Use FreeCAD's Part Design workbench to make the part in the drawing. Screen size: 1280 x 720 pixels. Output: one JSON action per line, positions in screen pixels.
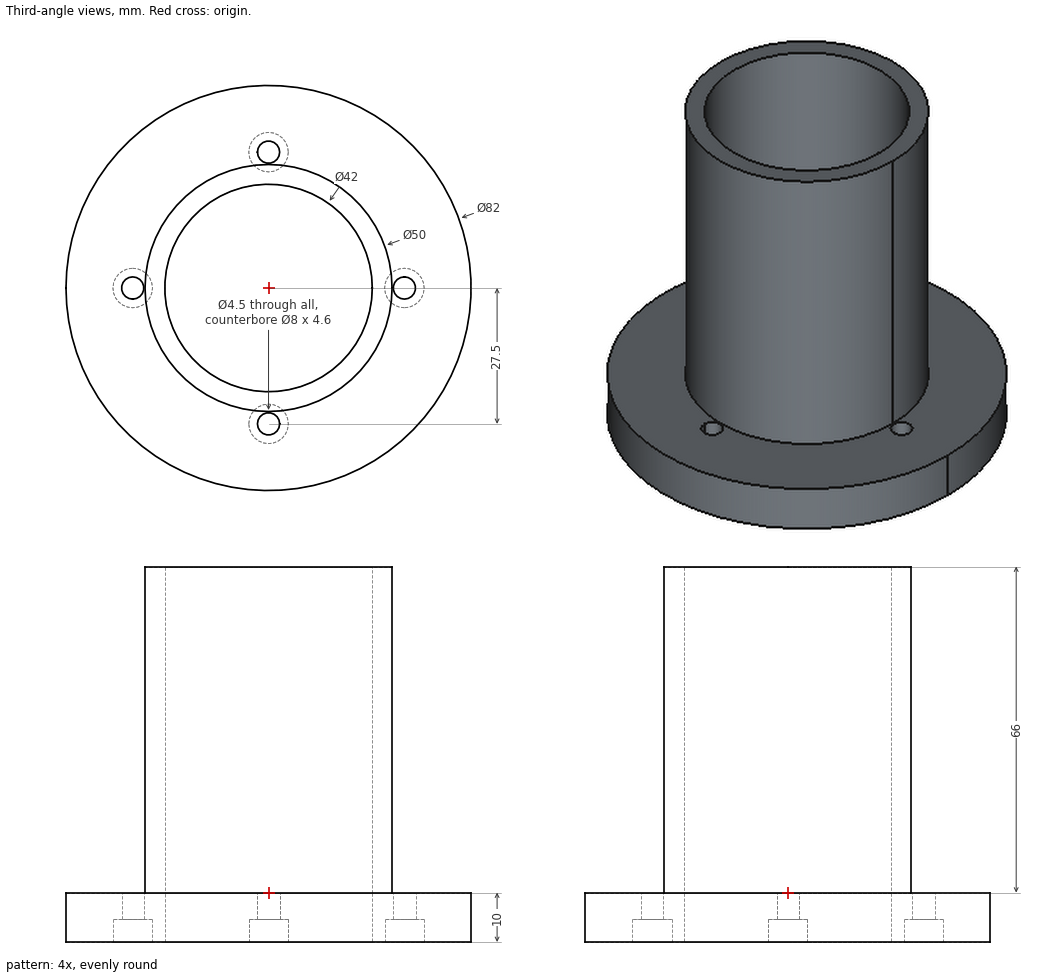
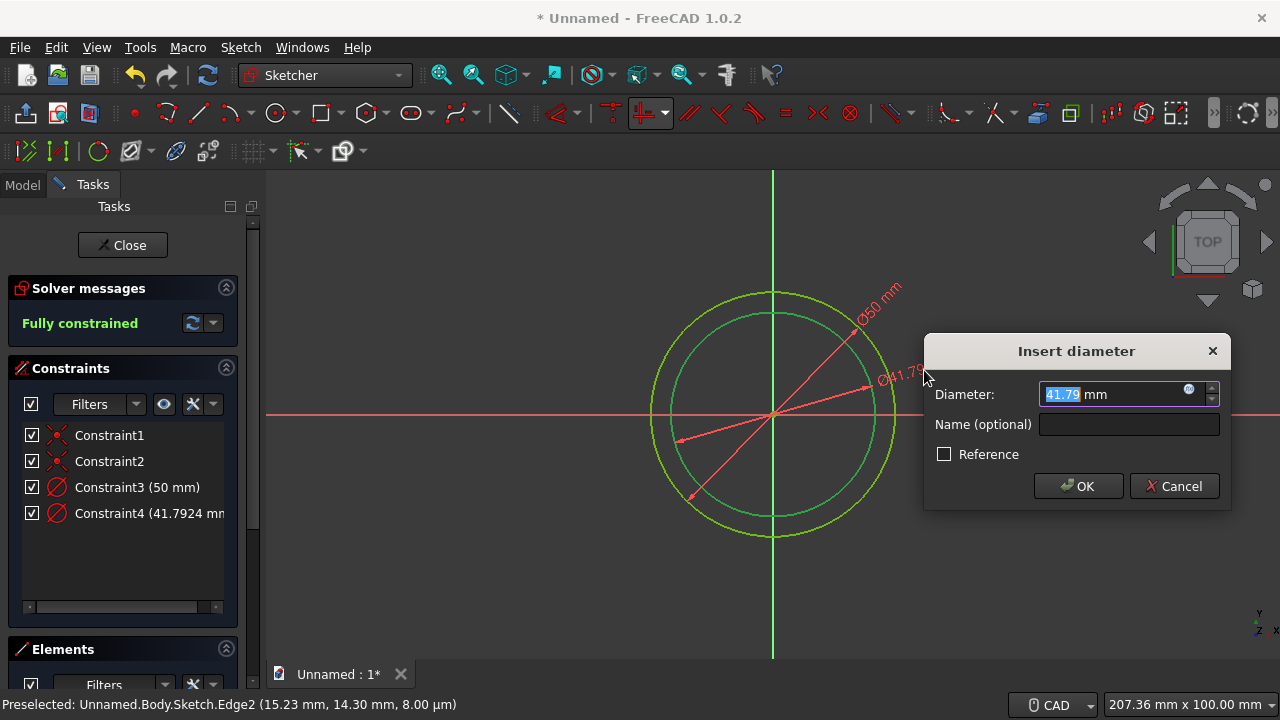
{"action": "type", "text": "42"}
{"action": "key", "text": "Return"}
{"action": "key", "text": "Escape"}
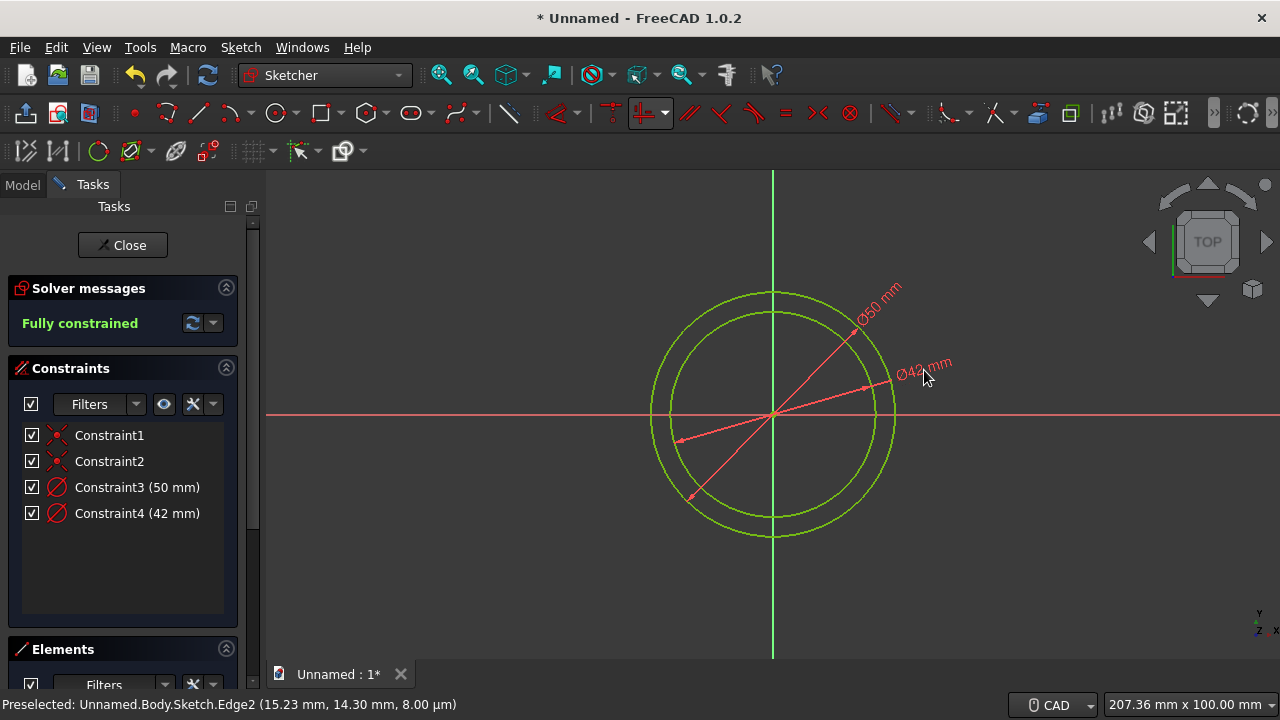
{"action": "left_click", "coordinate": [123, 245]}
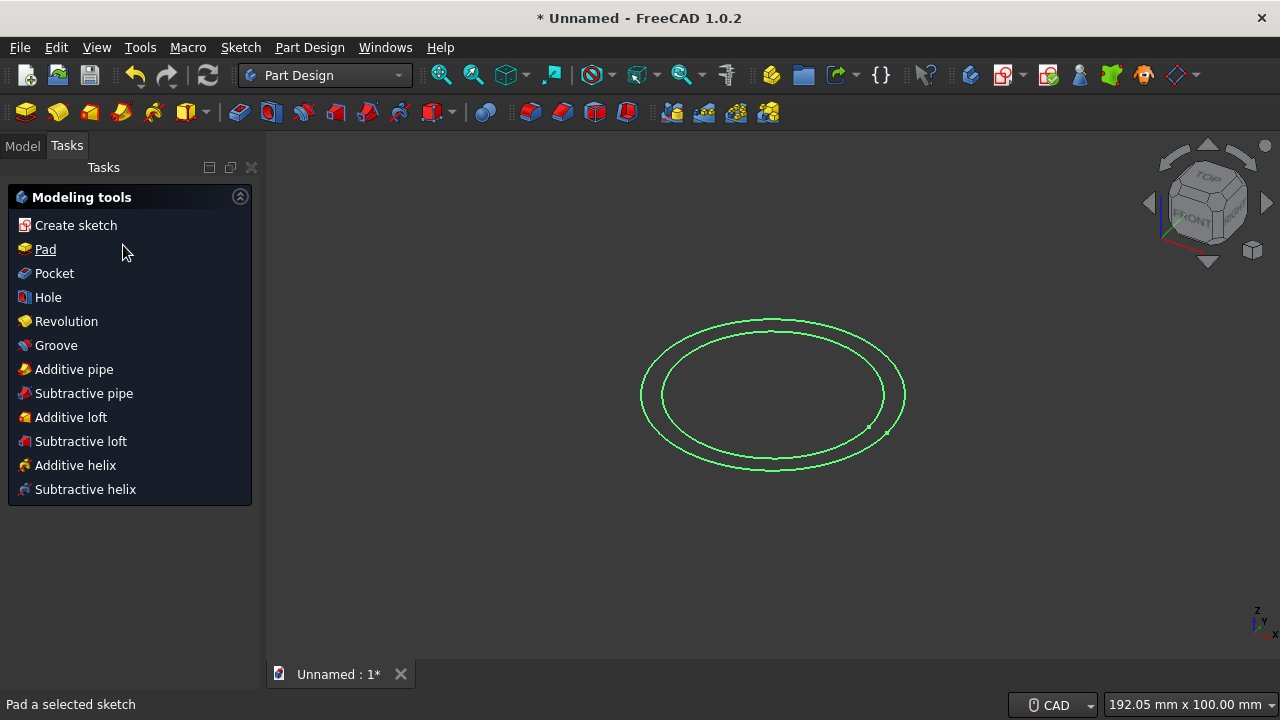
{"action": "left_click", "coordinate": [26, 112]}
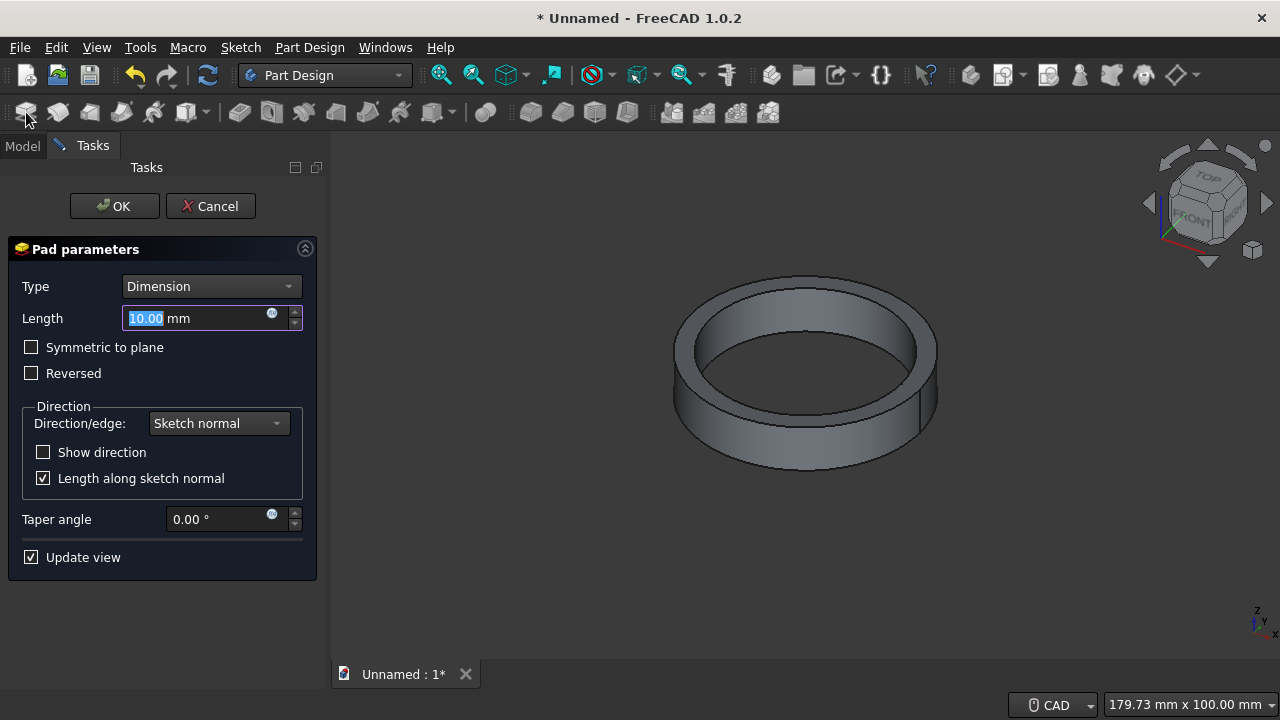
{"action": "type", "text": "66"}
{"action": "key", "text": "Tab"}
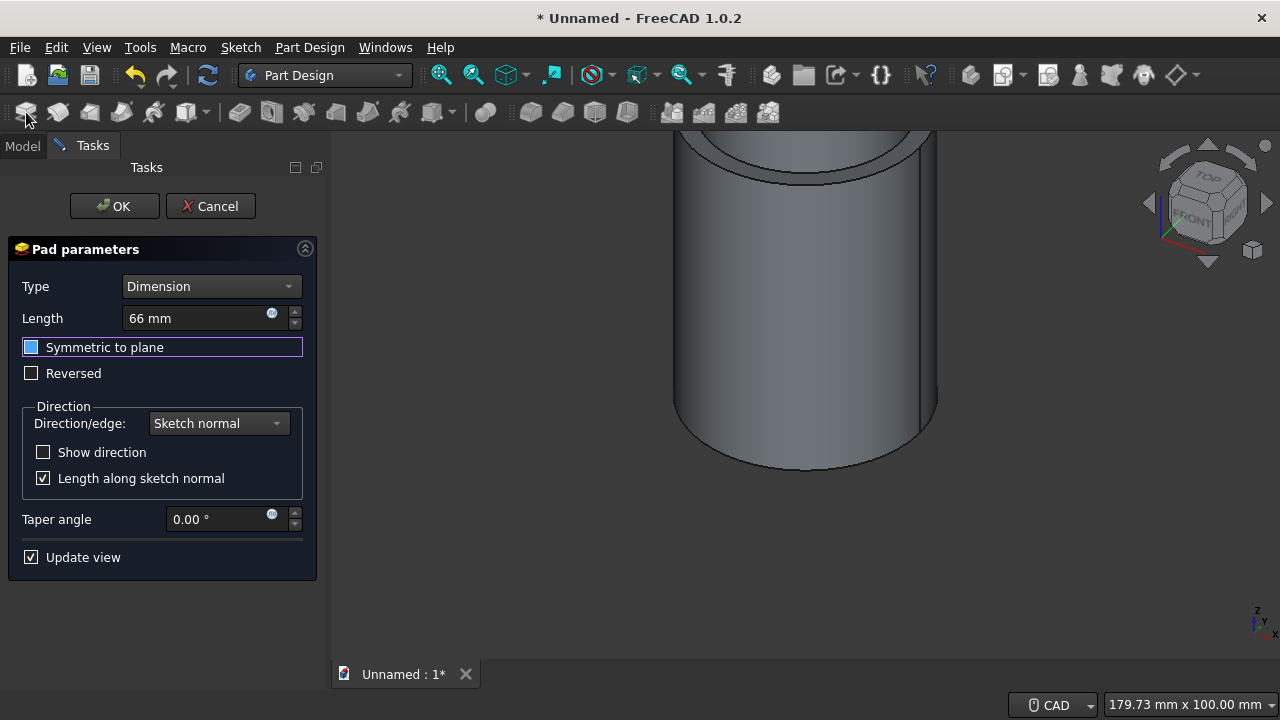
{"action": "left_click", "coordinate": [115, 206]}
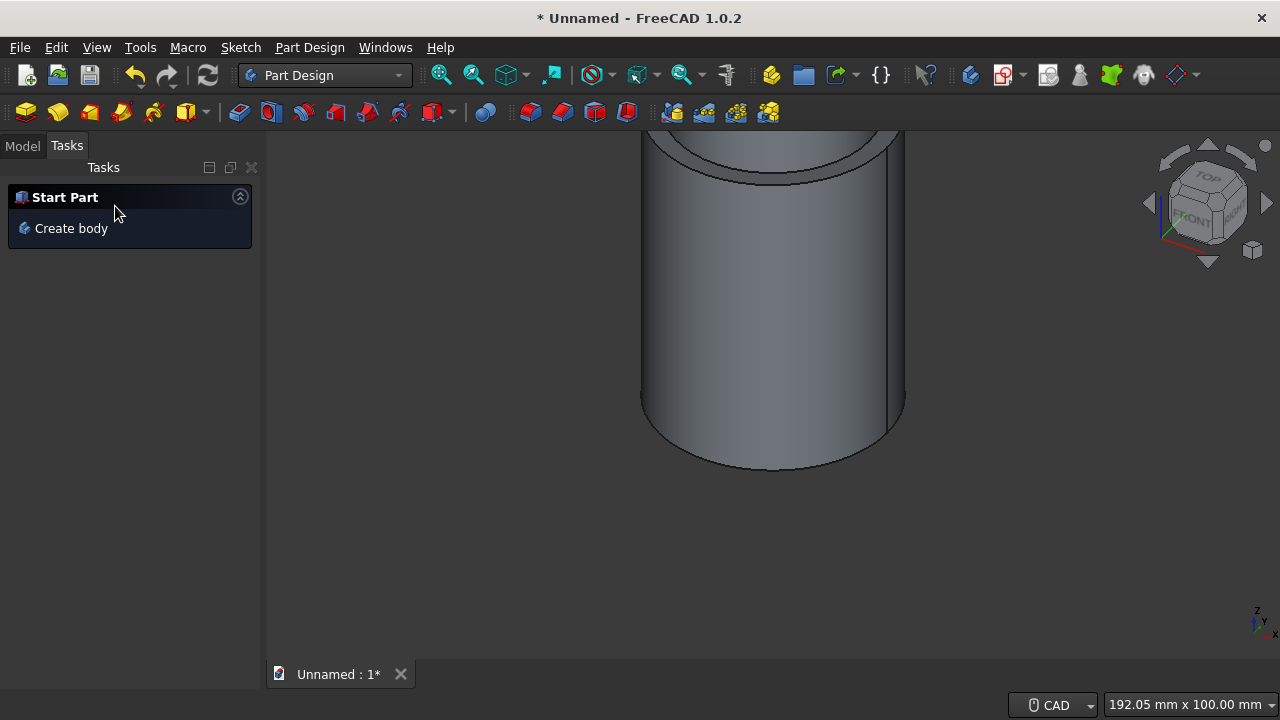
{"action": "left_click", "coordinate": [442, 76]}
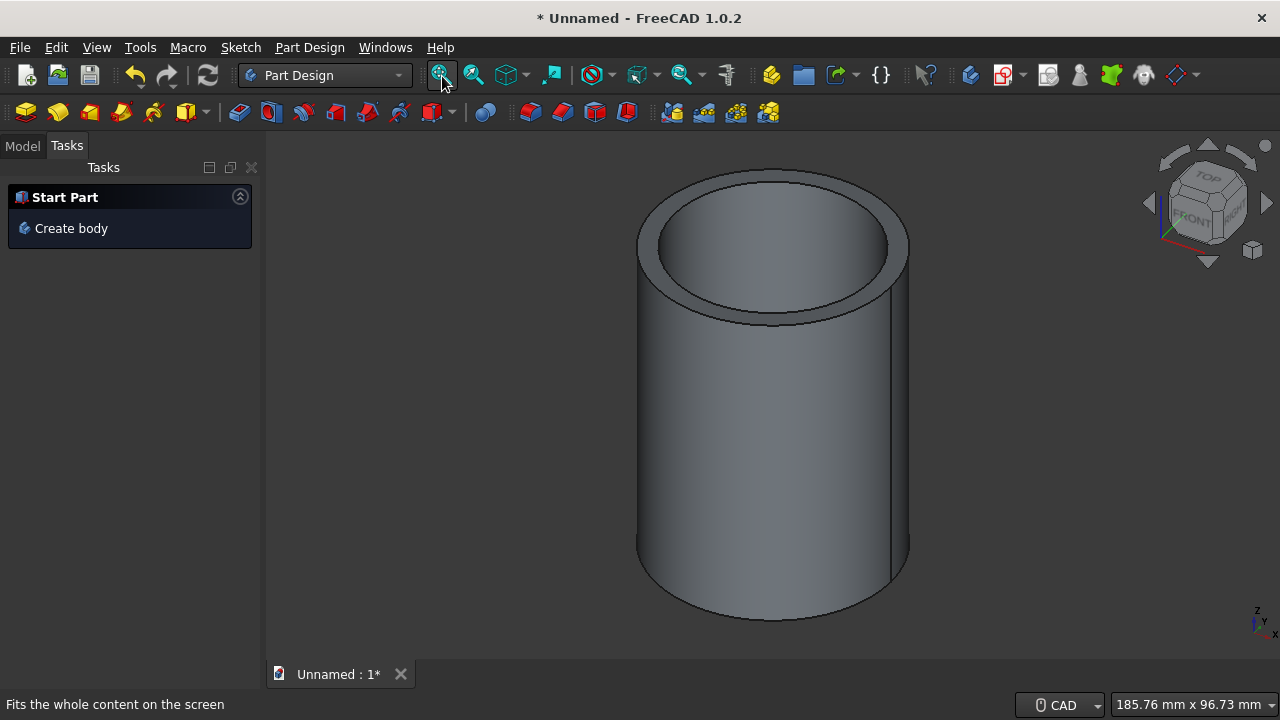
{"action": "left_click", "coordinate": [23, 145]}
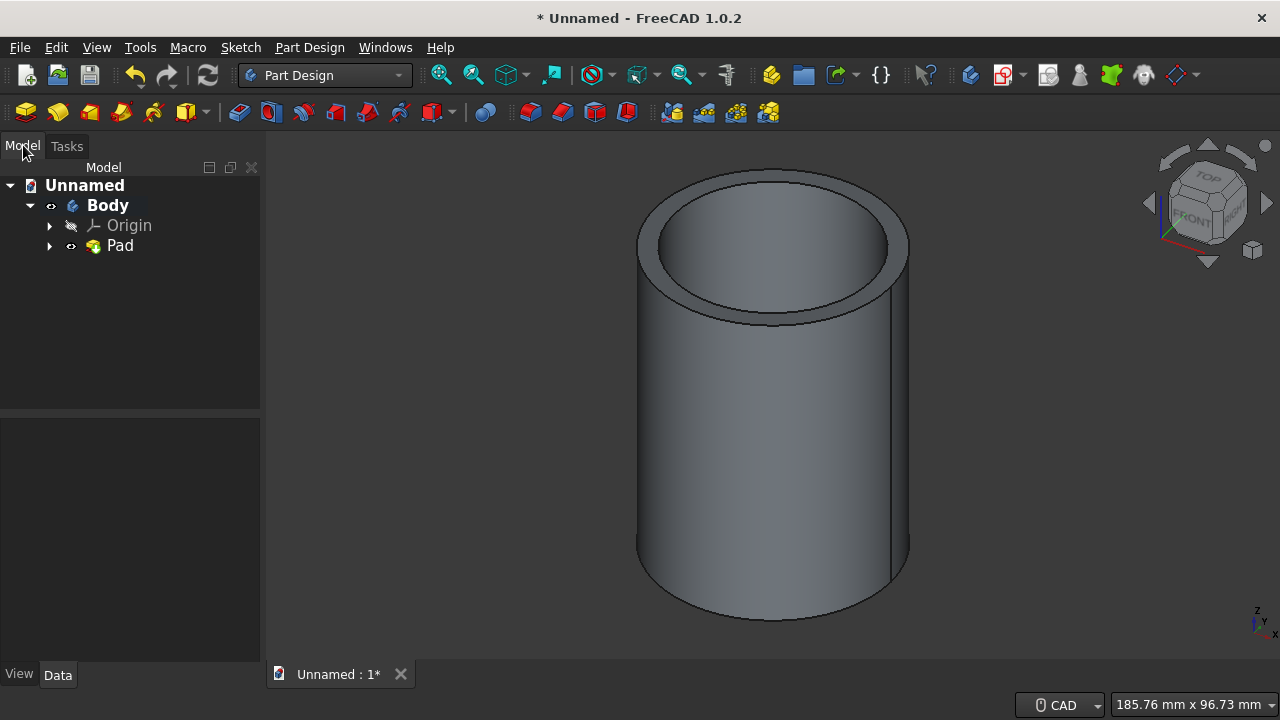
{"action": "left_click", "coordinate": [50, 226]}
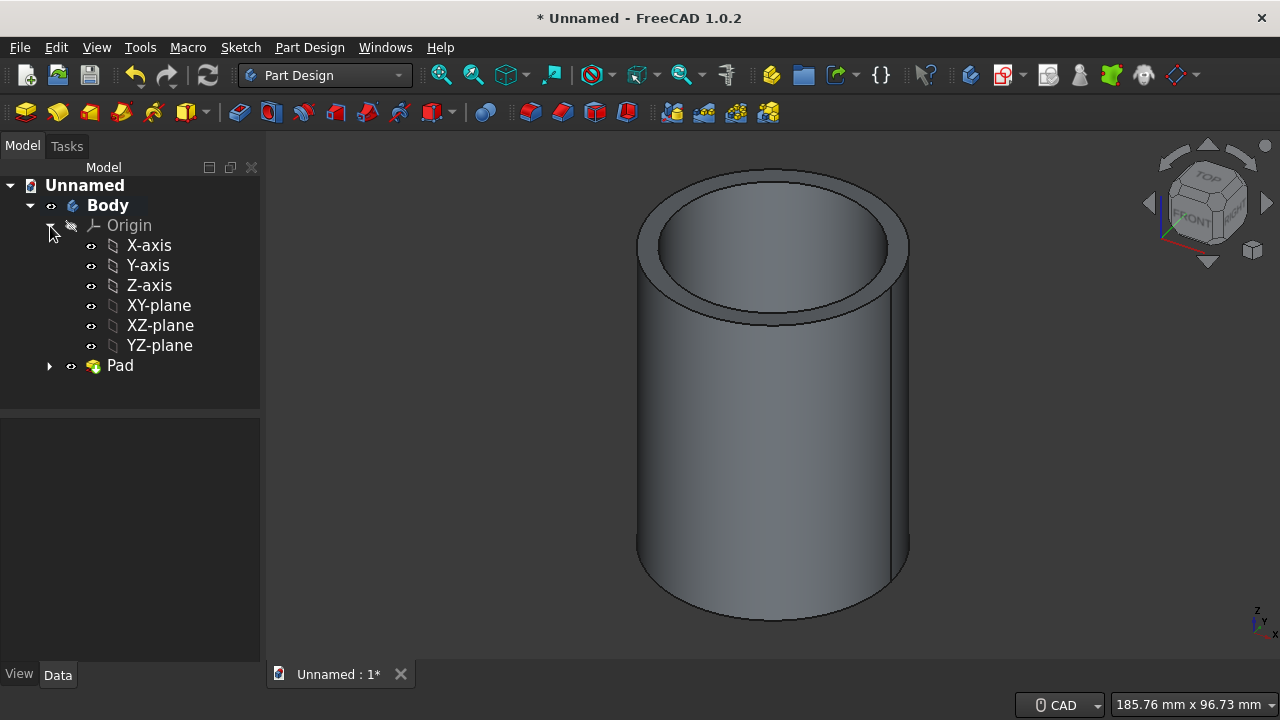
{"action": "left_click", "coordinate": [136, 306]}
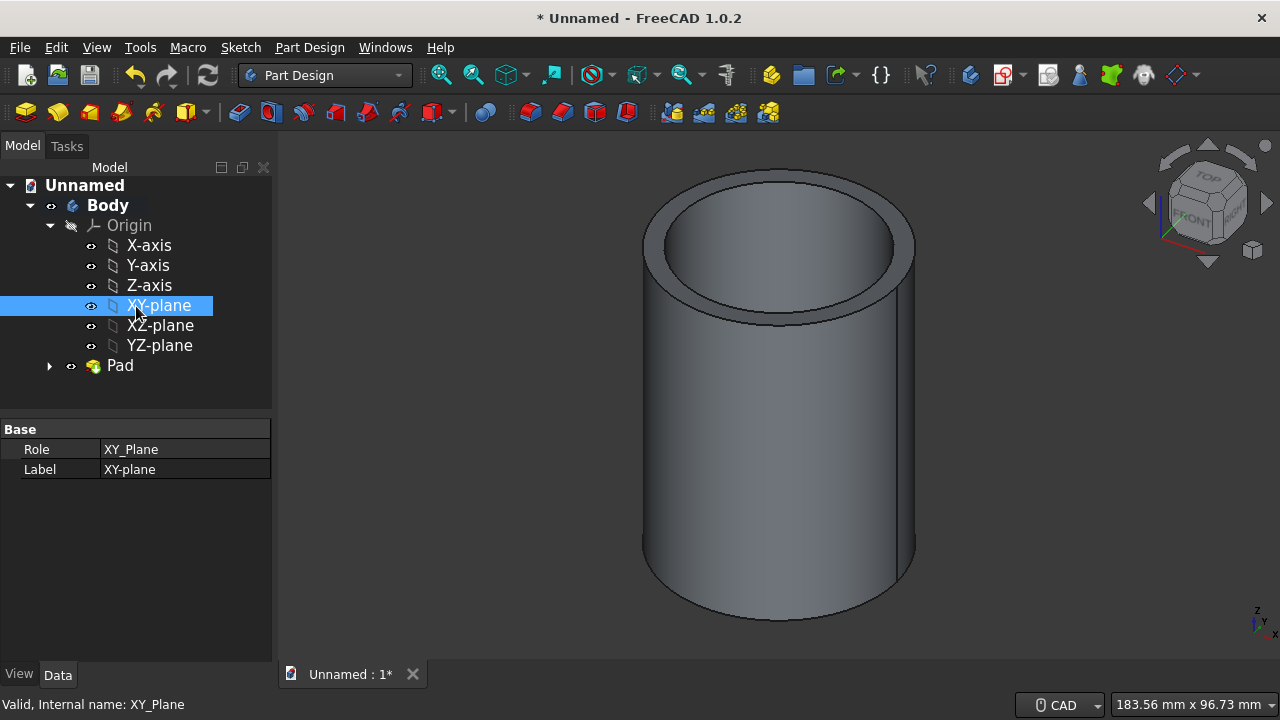
{"action": "left_click", "coordinate": [1176, 76]}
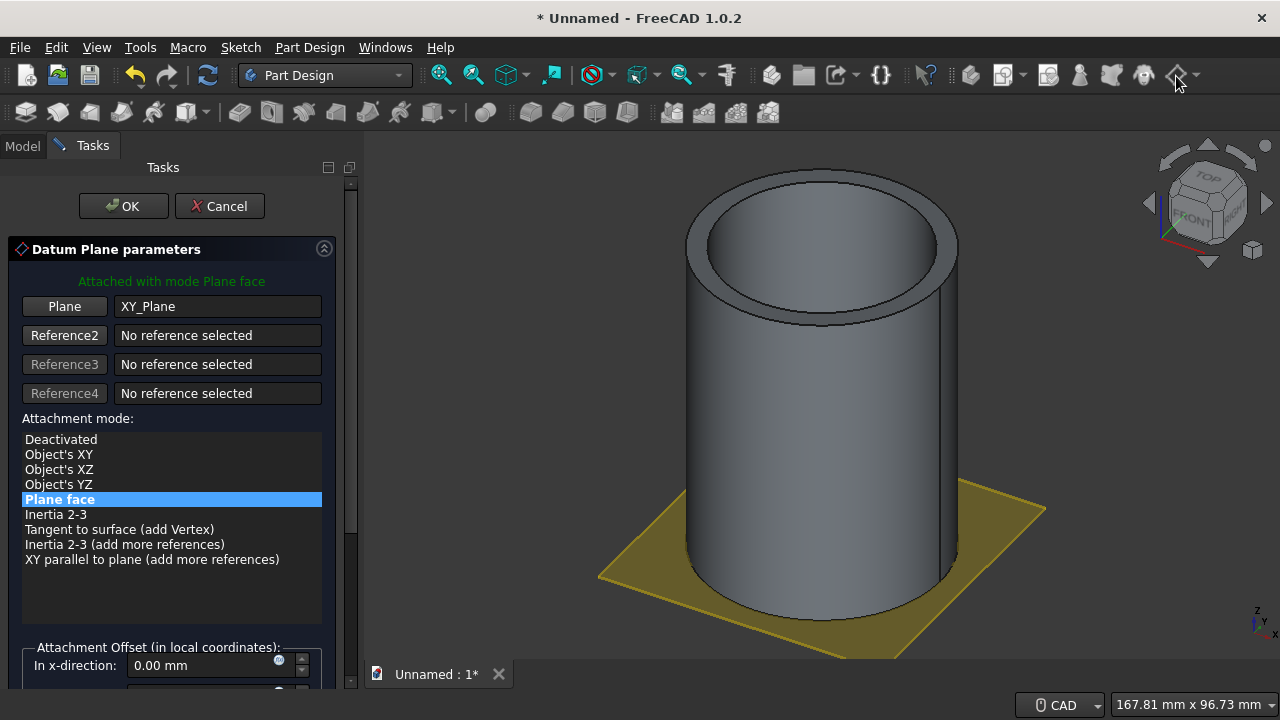
{"action": "scroll", "coordinate": [351, 432], "scroll_direction": "down", "scroll_amount": 2}